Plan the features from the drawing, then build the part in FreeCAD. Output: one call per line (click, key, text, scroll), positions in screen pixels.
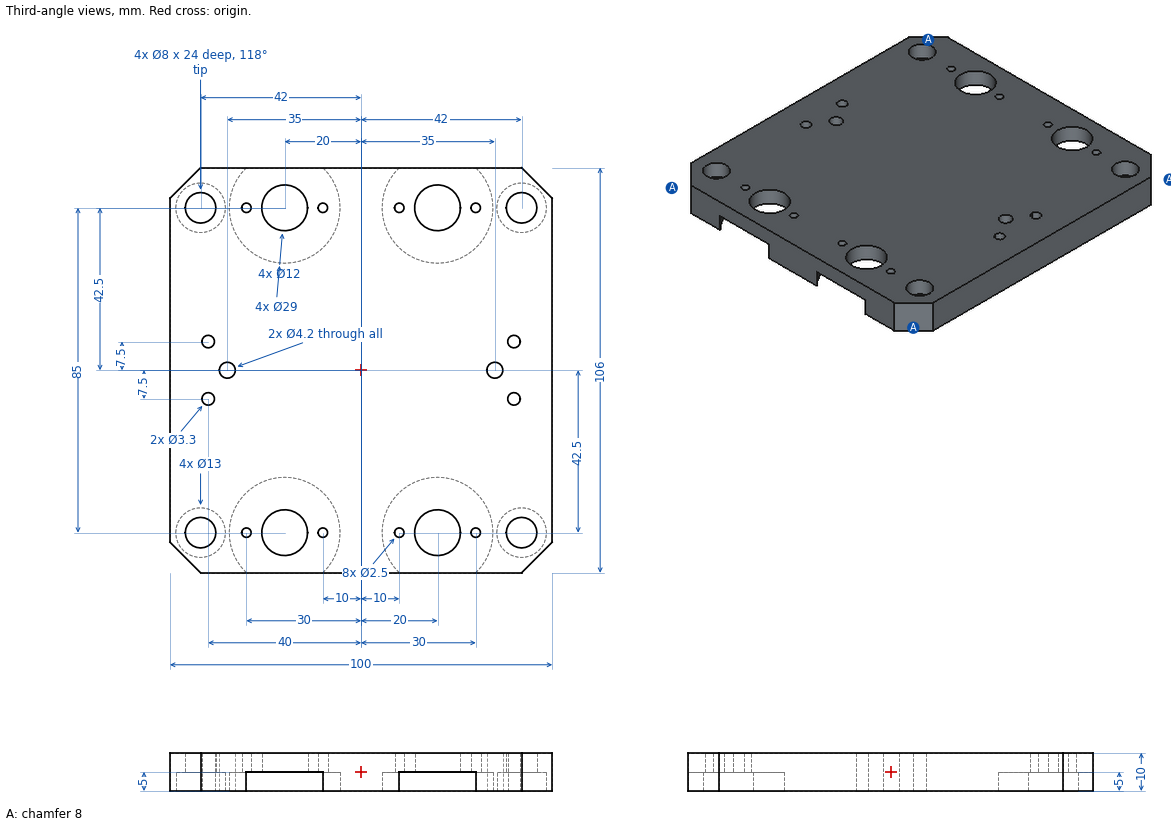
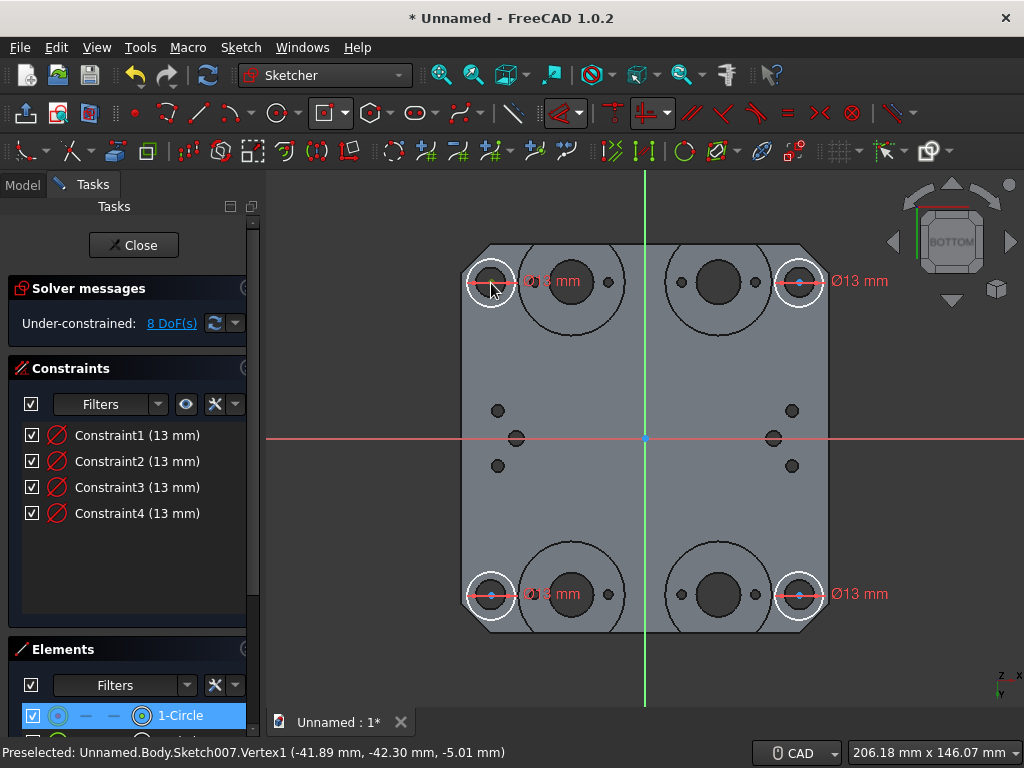
click(799, 283)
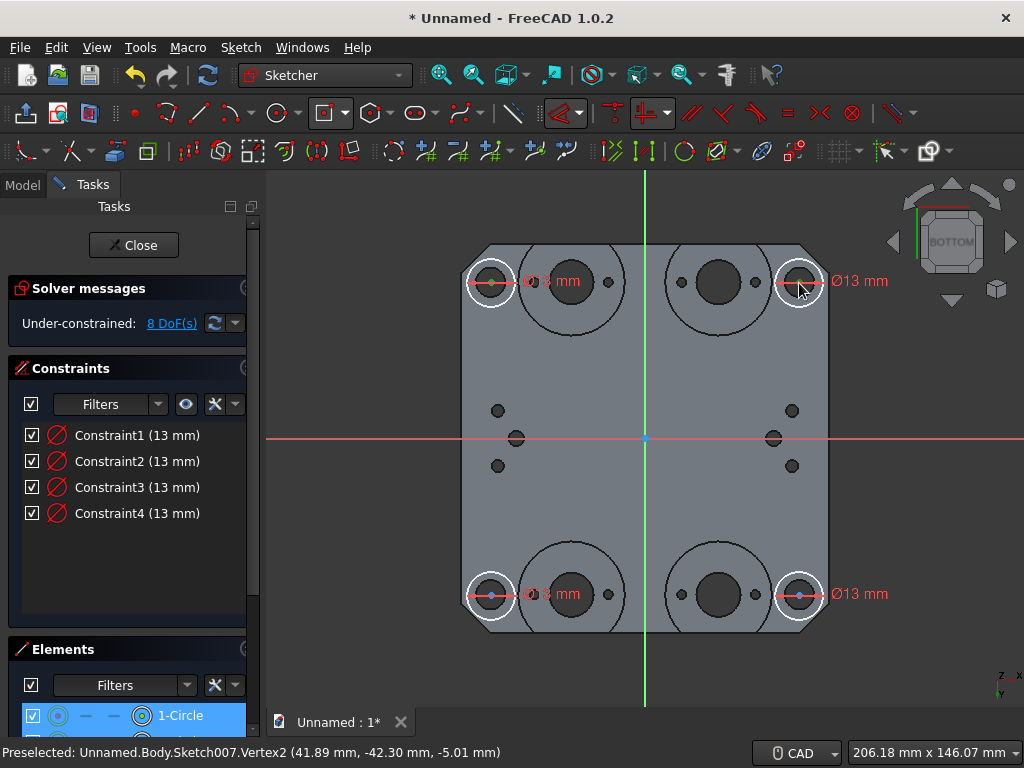
click(670, 114)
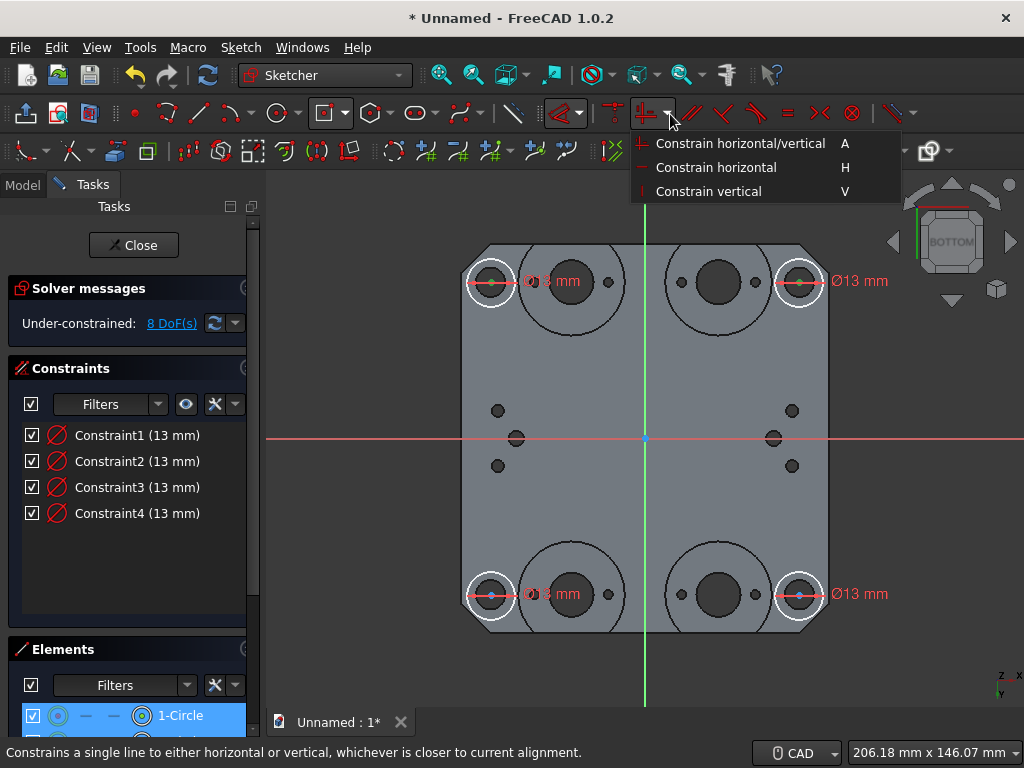
click(766, 167)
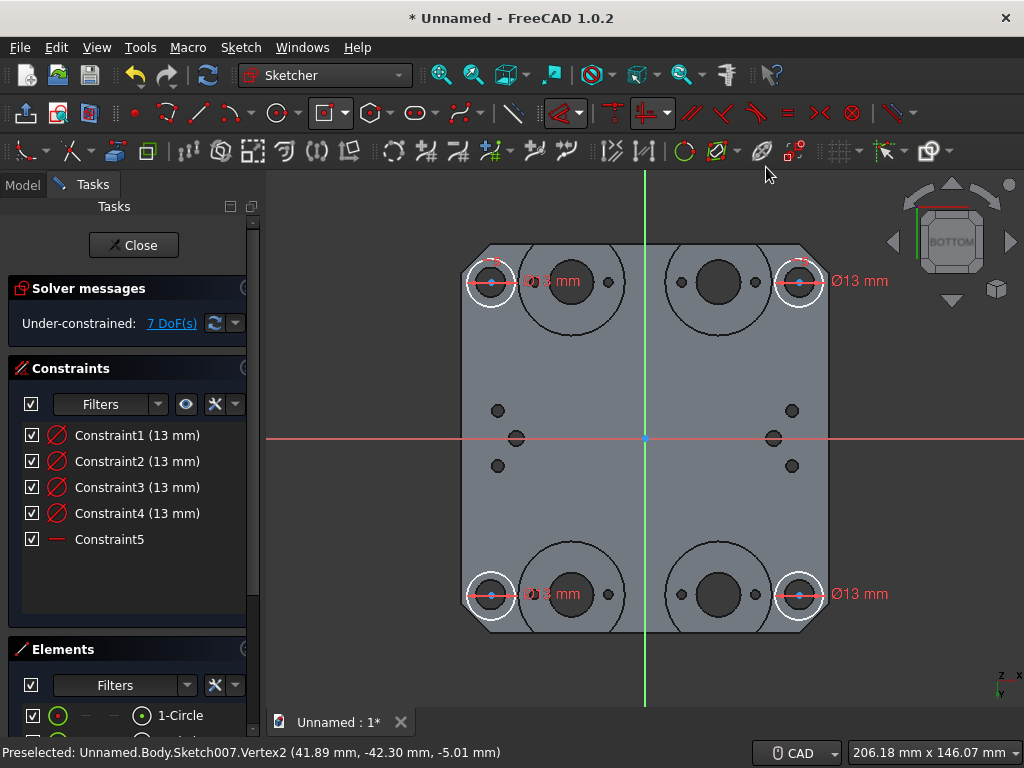
click(491, 283)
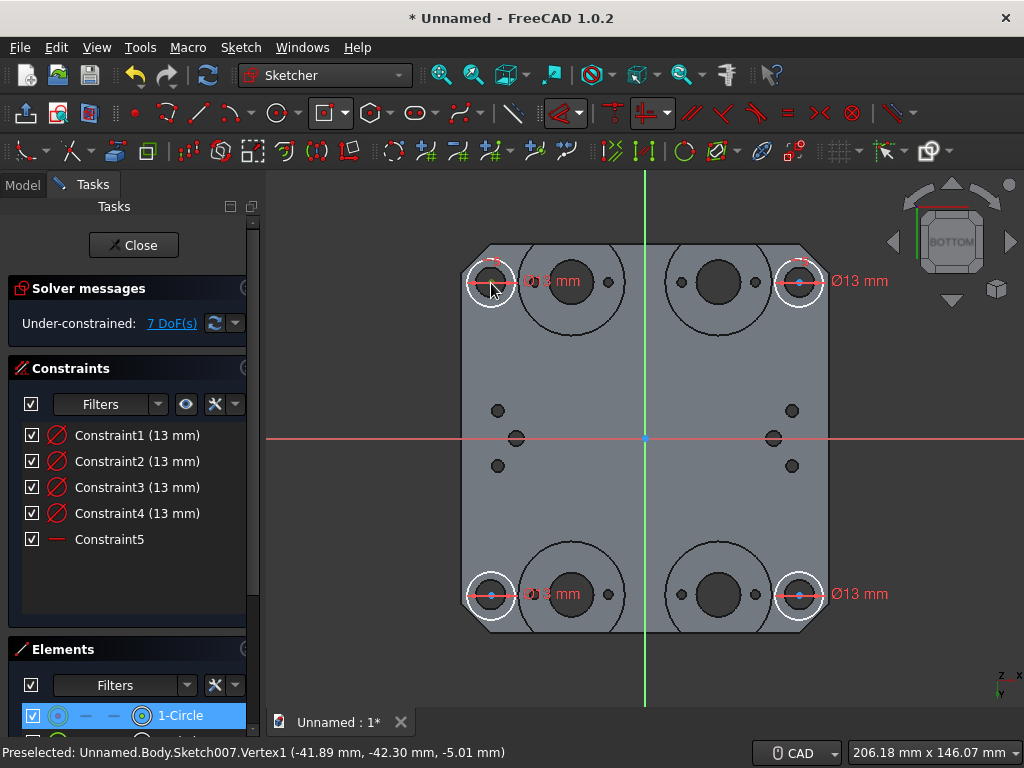
click(491, 596)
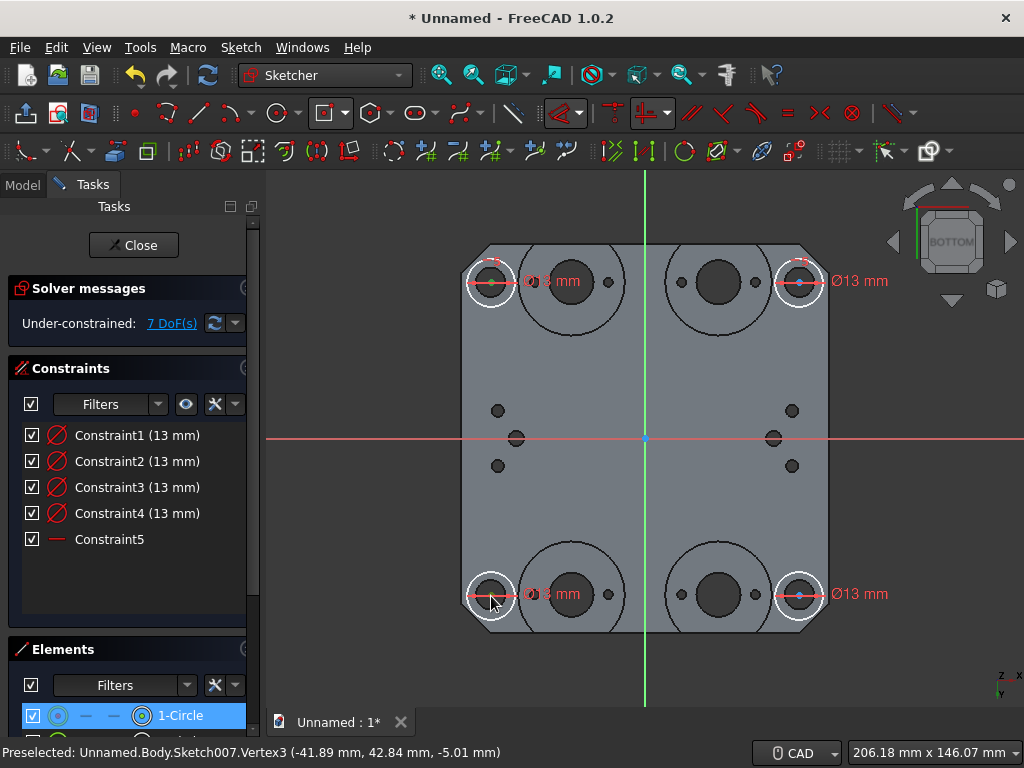
click(670, 114)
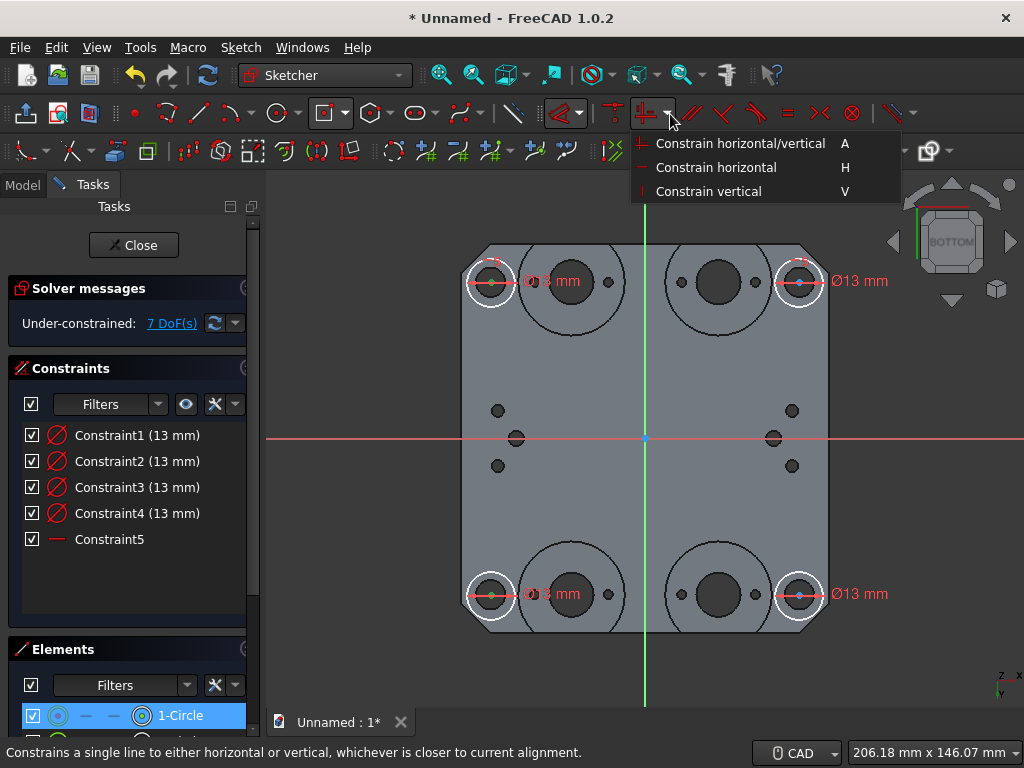
click(766, 191)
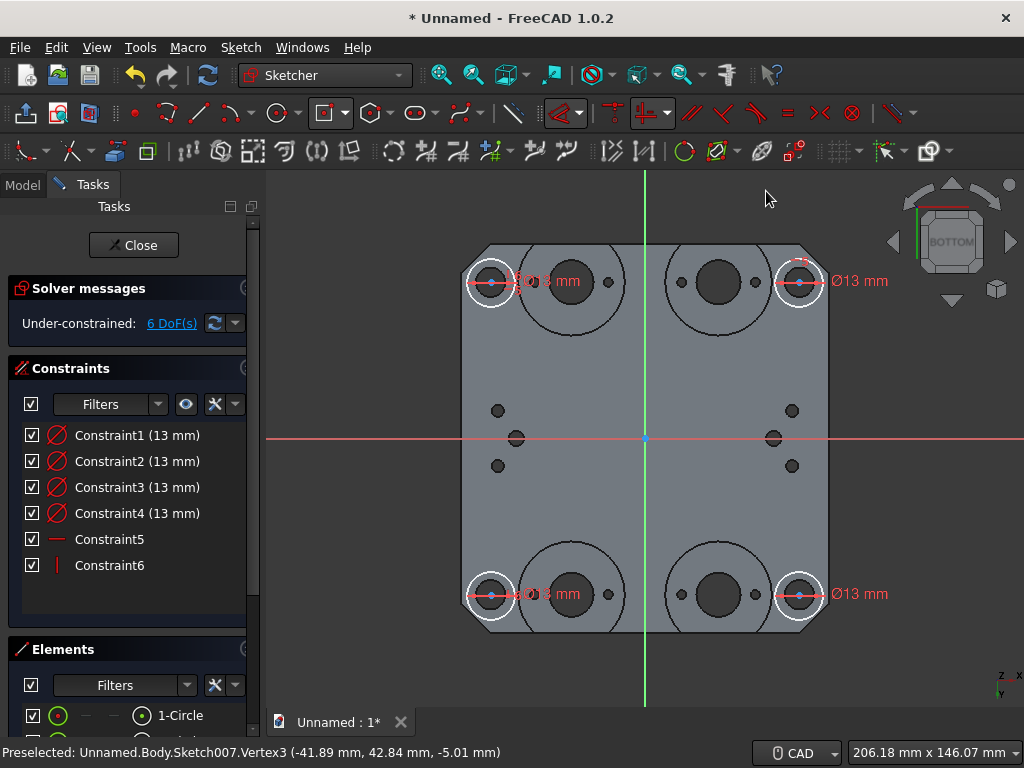
click(799, 283)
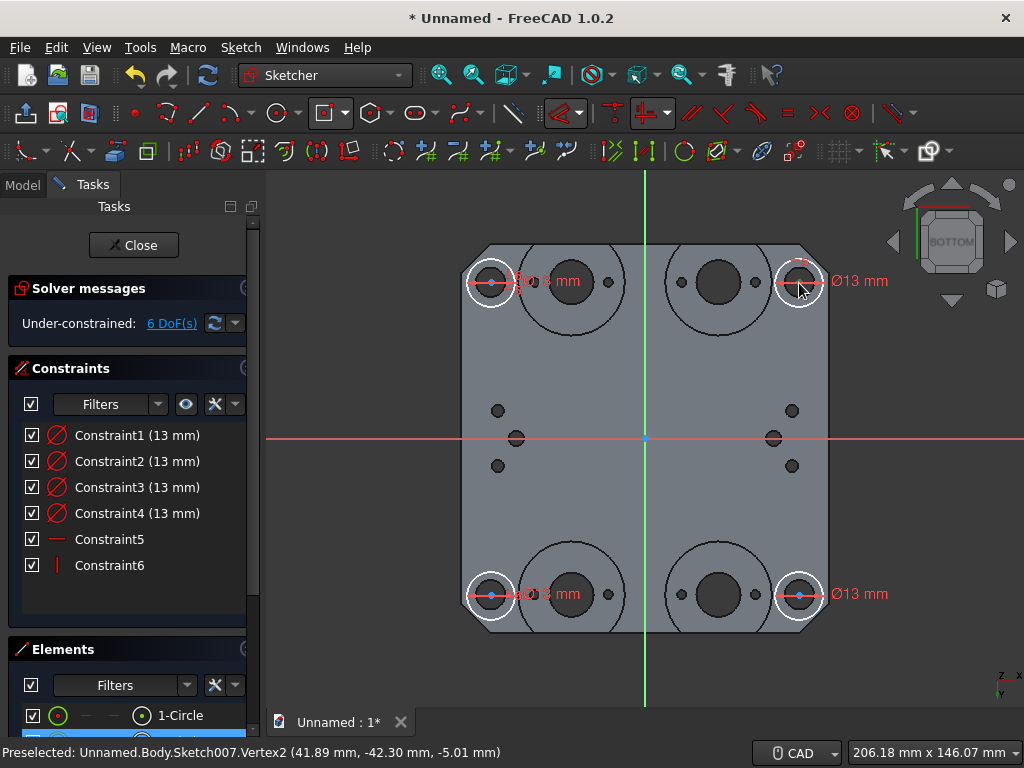
click(799, 596)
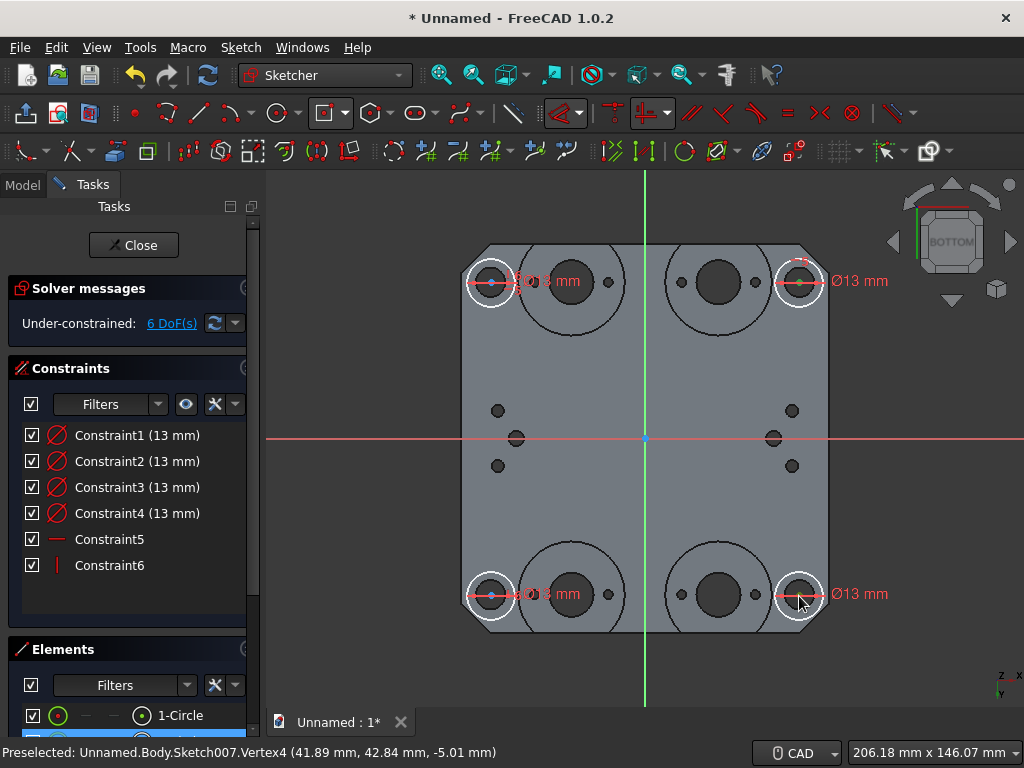
click(670, 114)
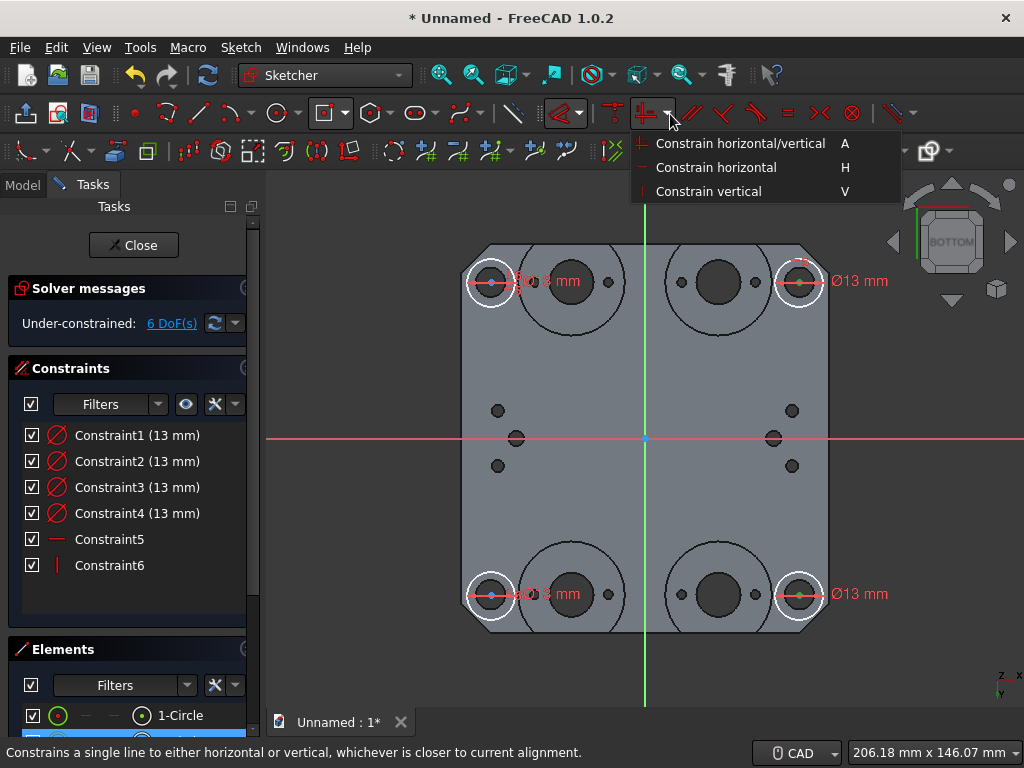
click(766, 191)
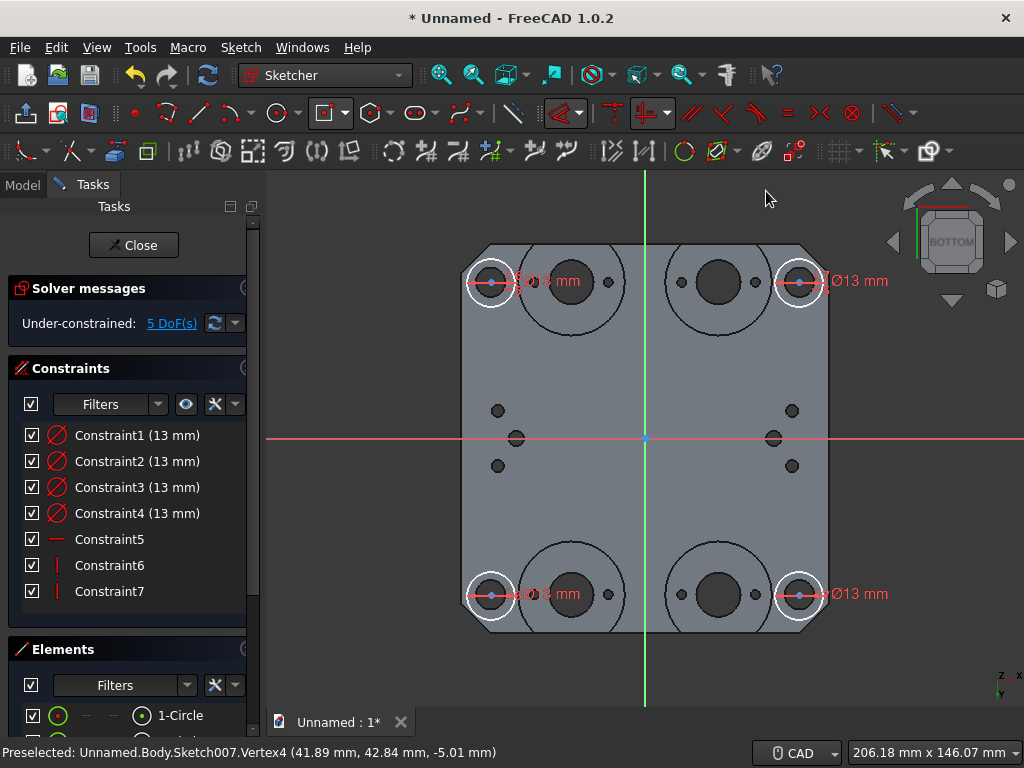
click(491, 596)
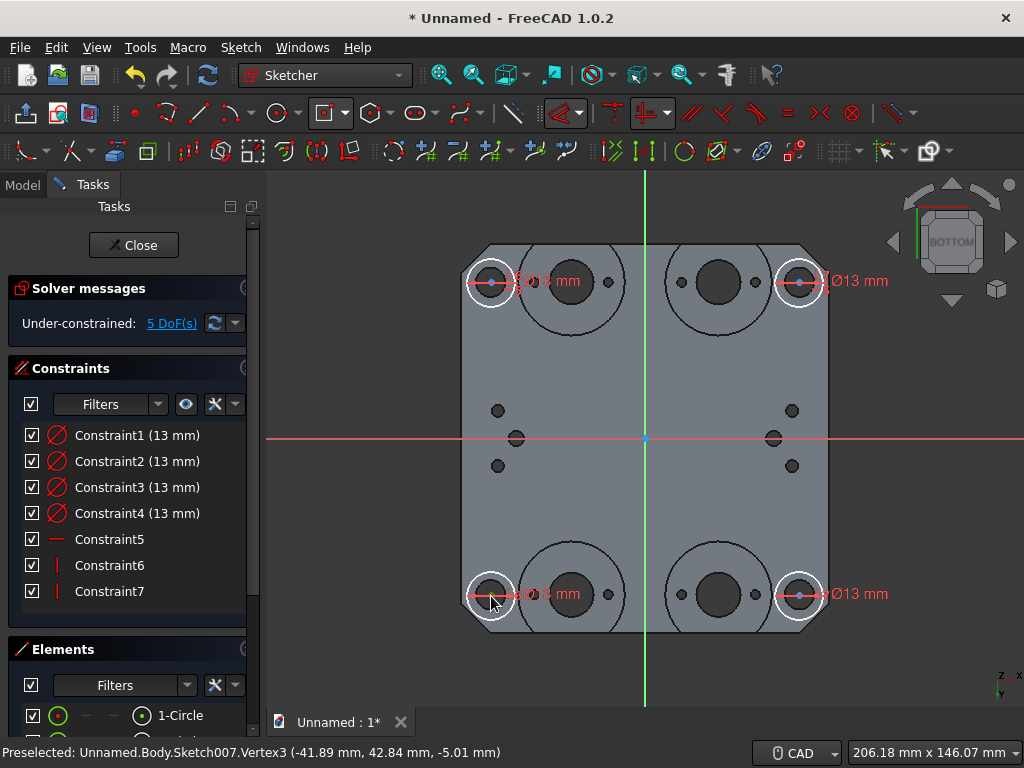
click(799, 596)